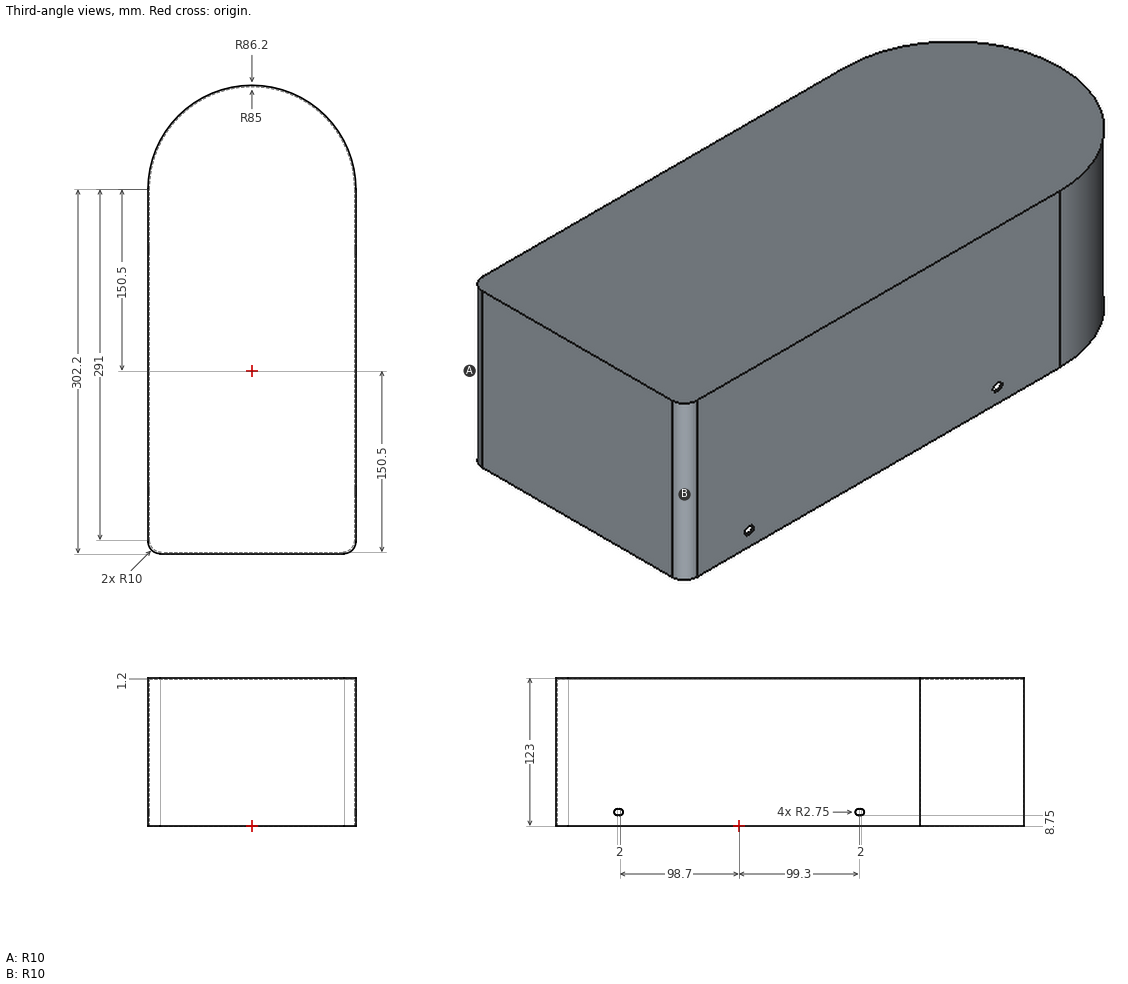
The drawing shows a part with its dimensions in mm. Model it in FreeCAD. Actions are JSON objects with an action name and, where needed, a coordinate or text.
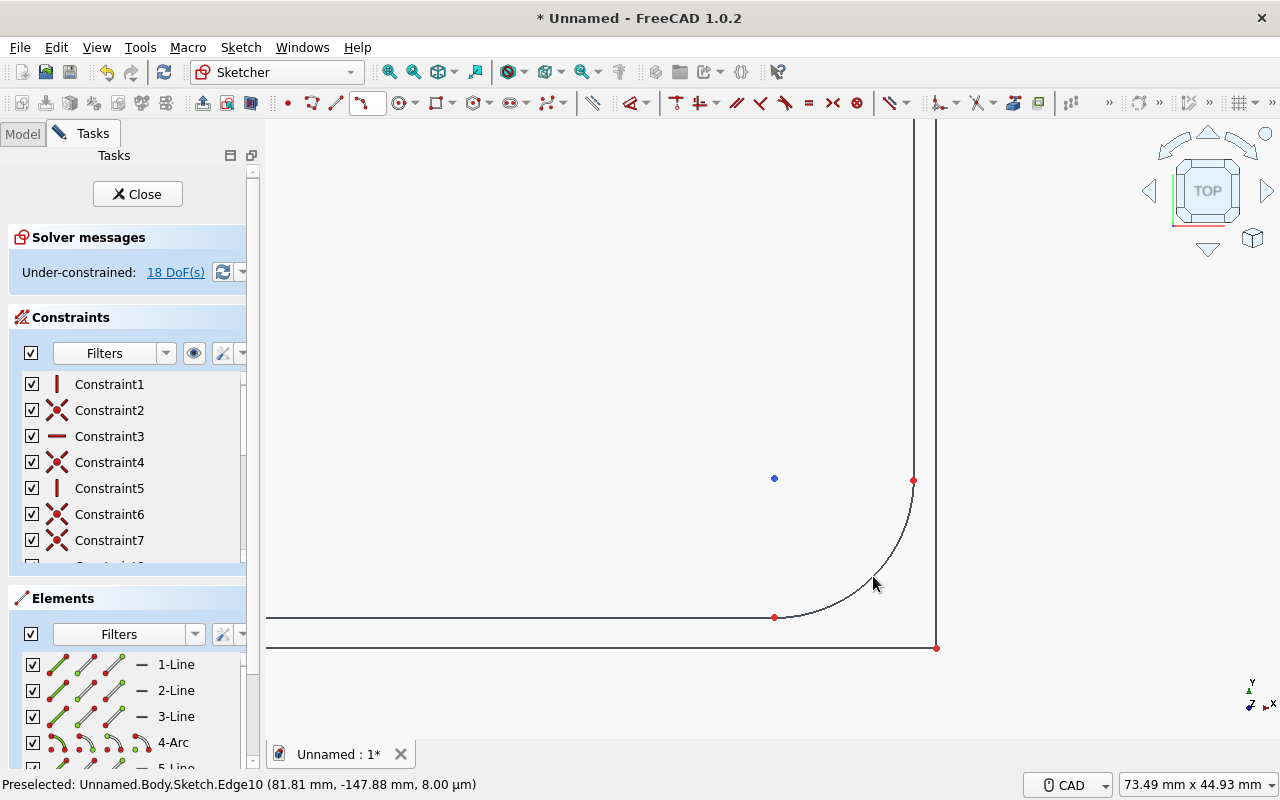
{"action": "left_click", "coordinate": [361, 618]}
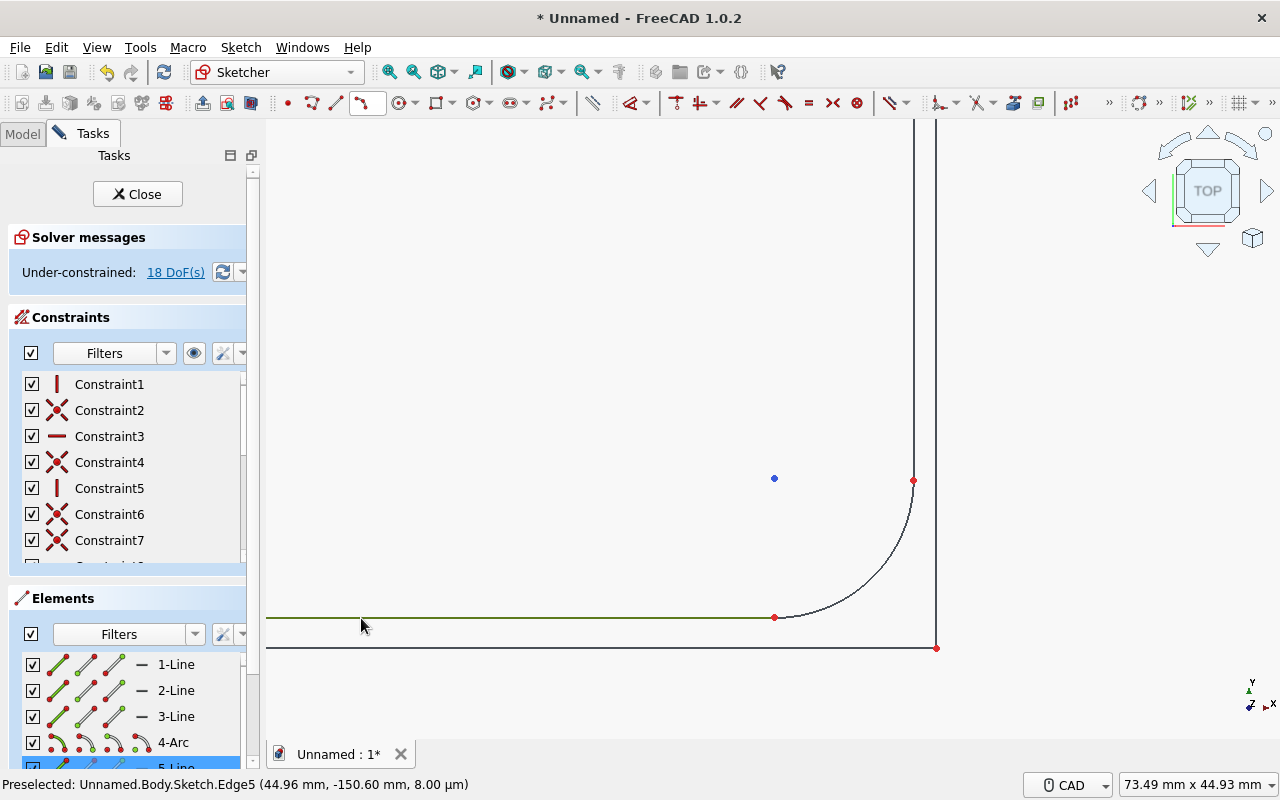
{"action": "scroll", "coordinate": [782, 628], "scroll_direction": "down", "scroll_amount": 13}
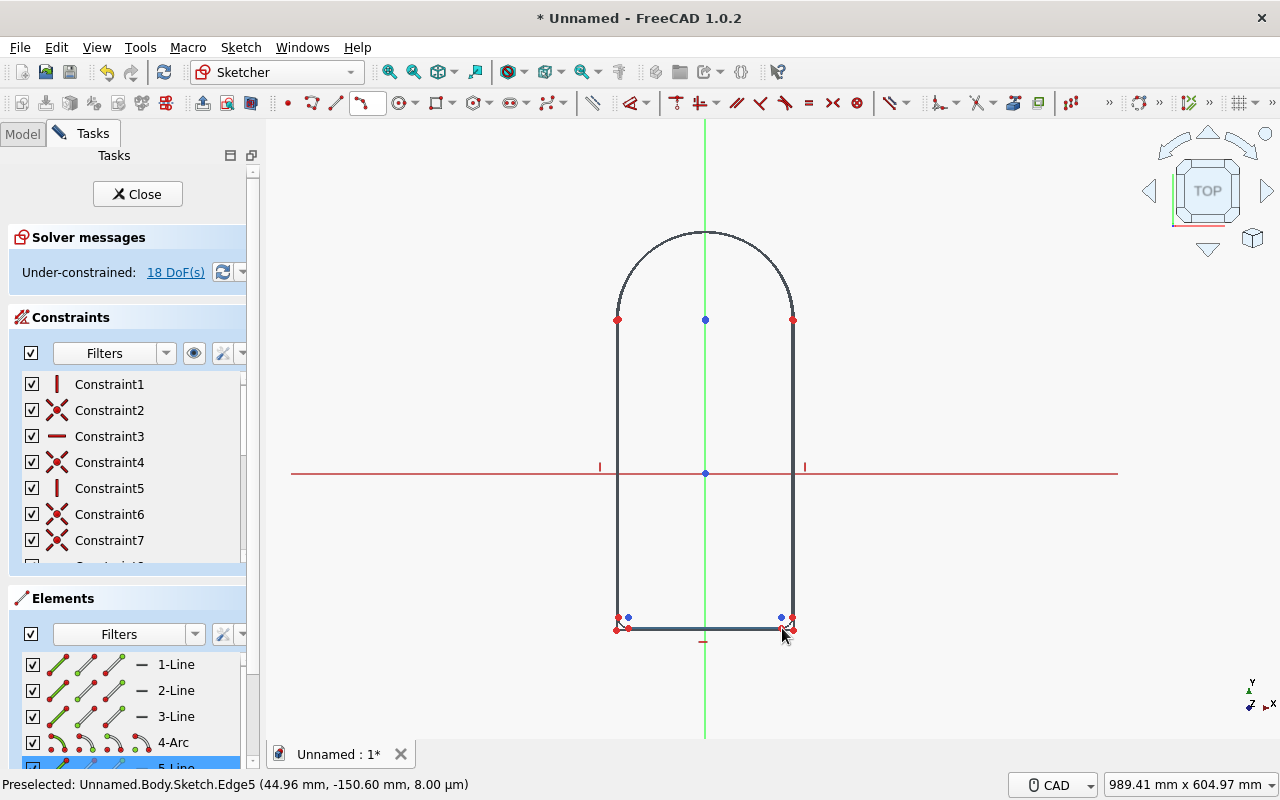
{"action": "scroll", "coordinate": [619, 622], "scroll_direction": "up", "scroll_amount": 9}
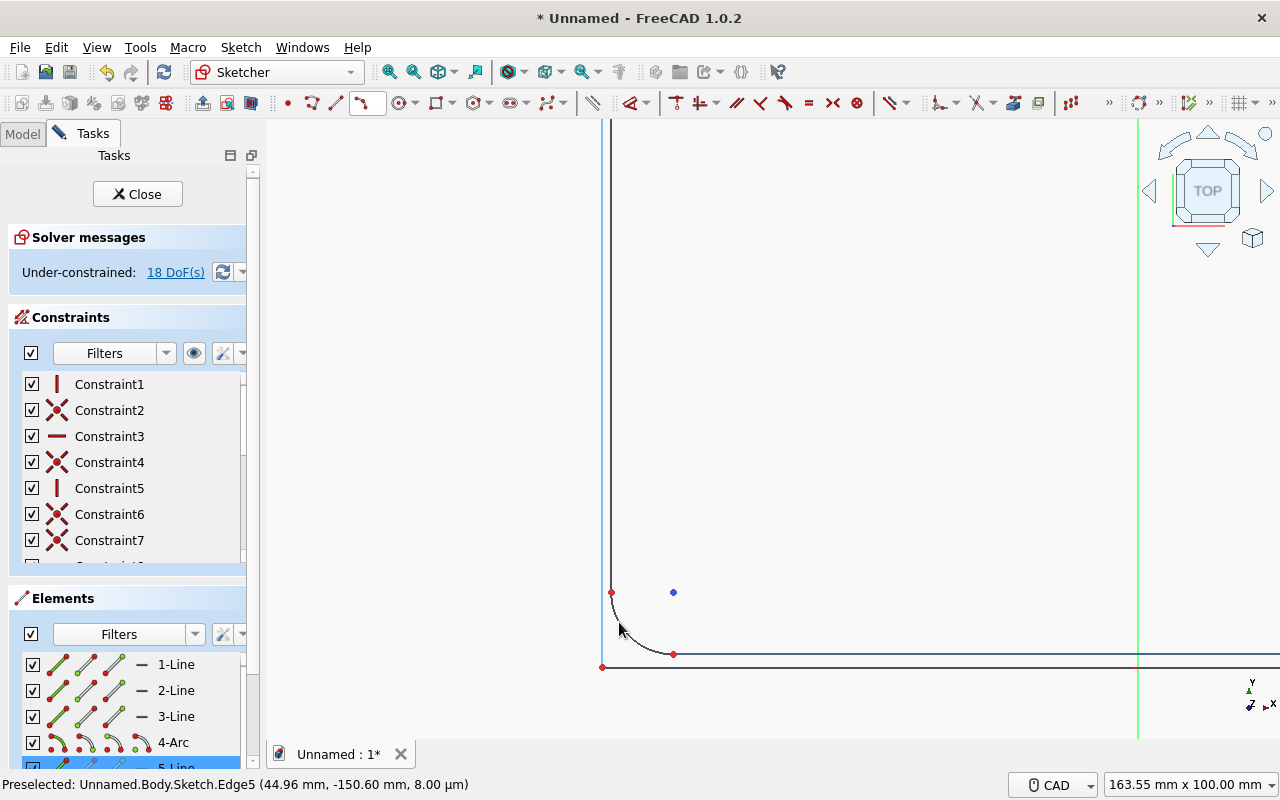
{"action": "left_click", "coordinate": [618, 620]}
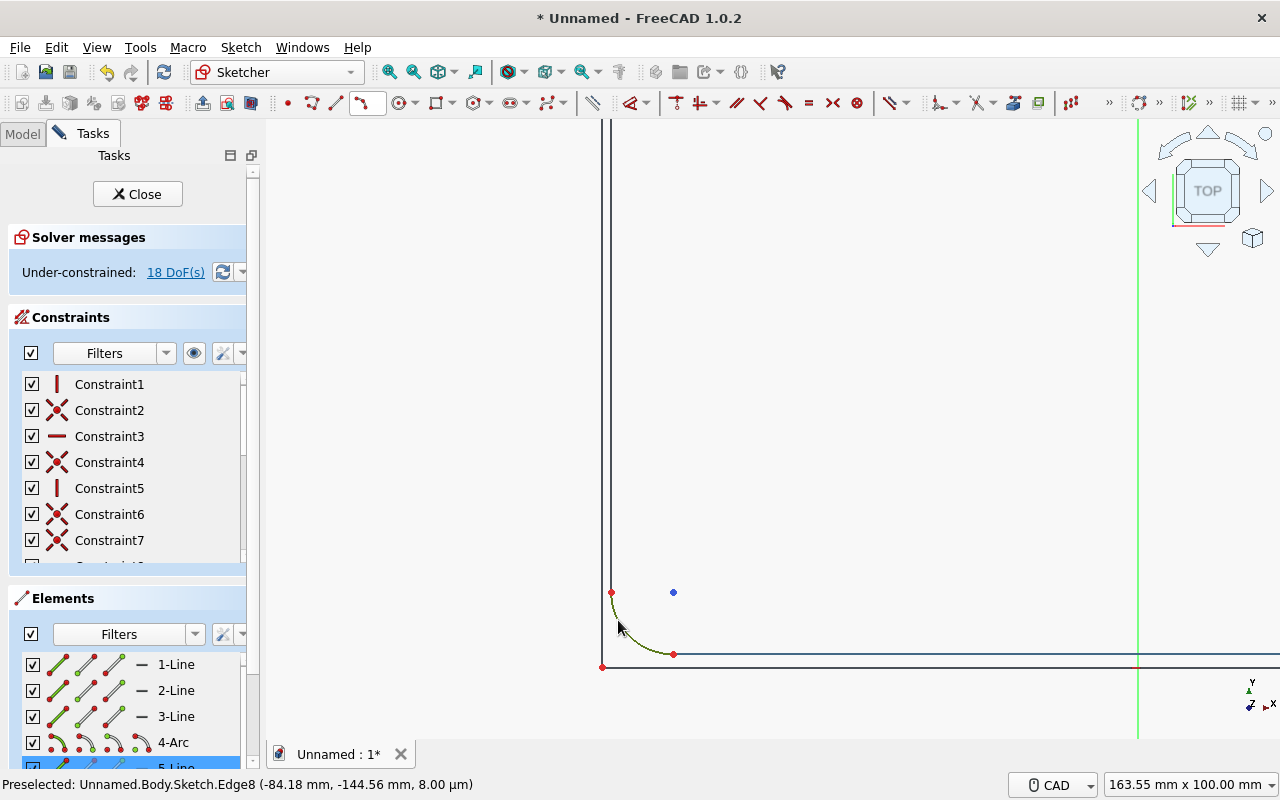
{"action": "key", "text": "t"}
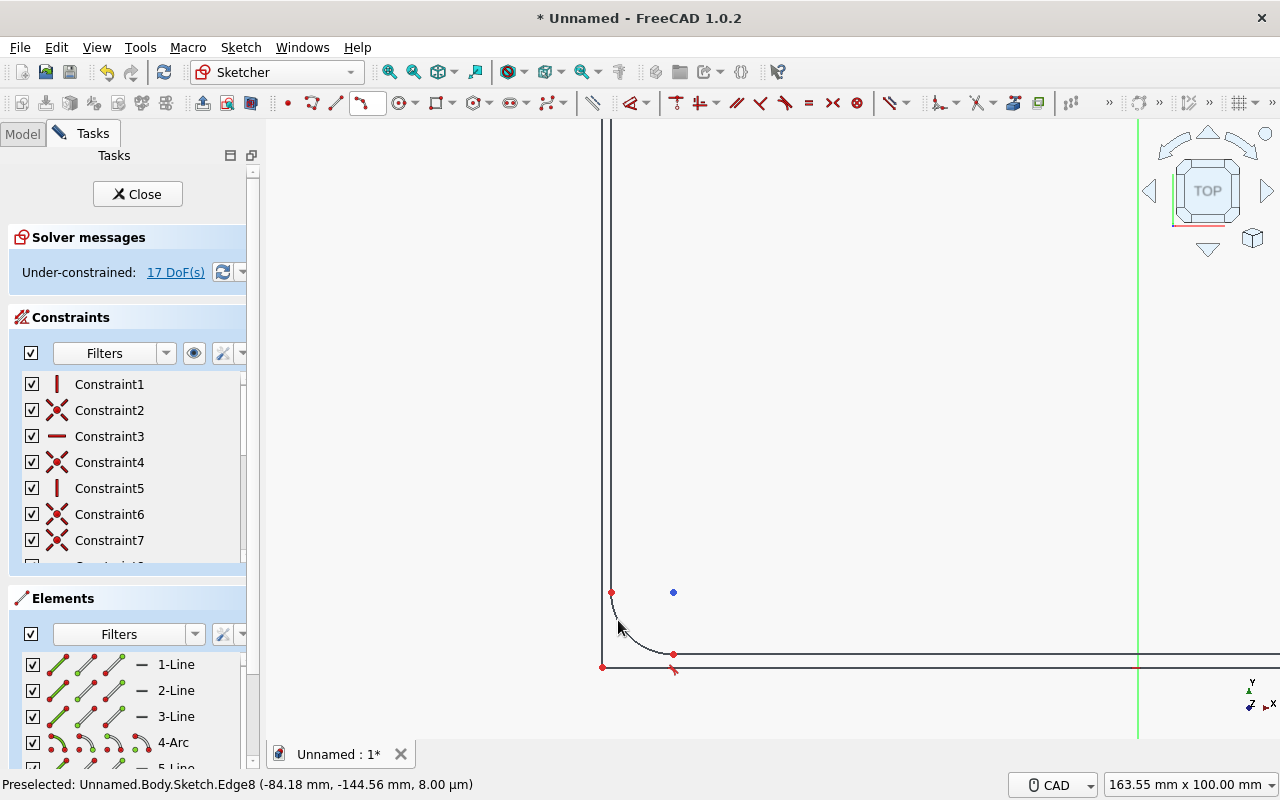
{"action": "left_click", "coordinate": [952, 654]}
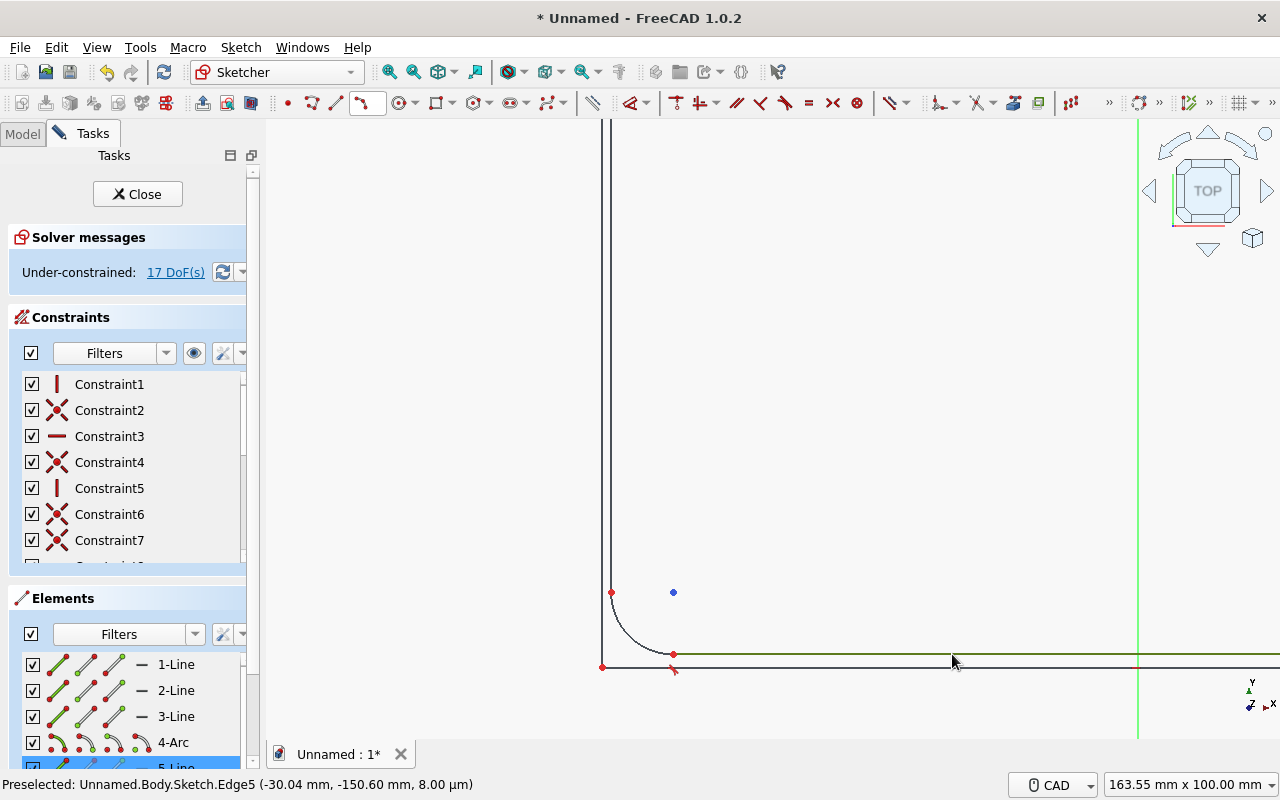
{"action": "scroll", "coordinate": [619, 621], "scroll_direction": "down", "scroll_amount": 9}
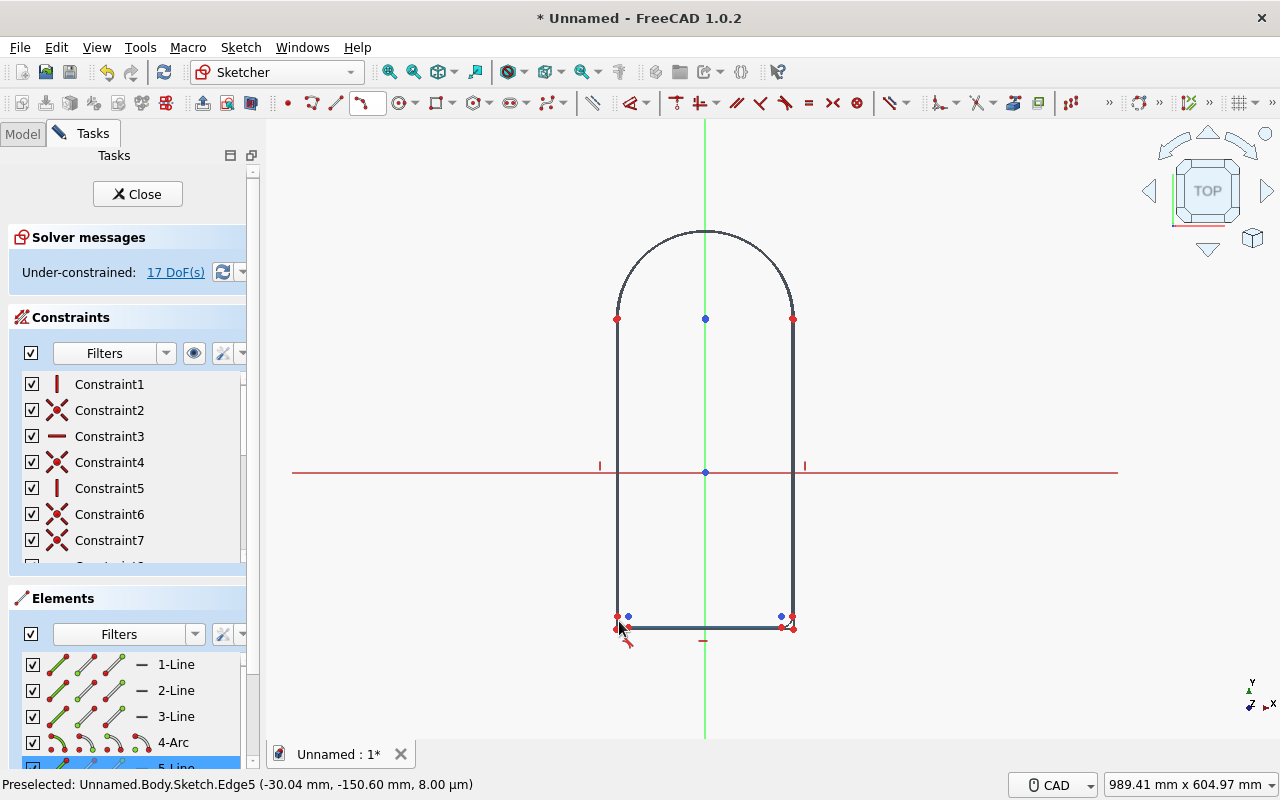
{"action": "scroll", "coordinate": [787, 626], "scroll_direction": "up", "scroll_amount": 8}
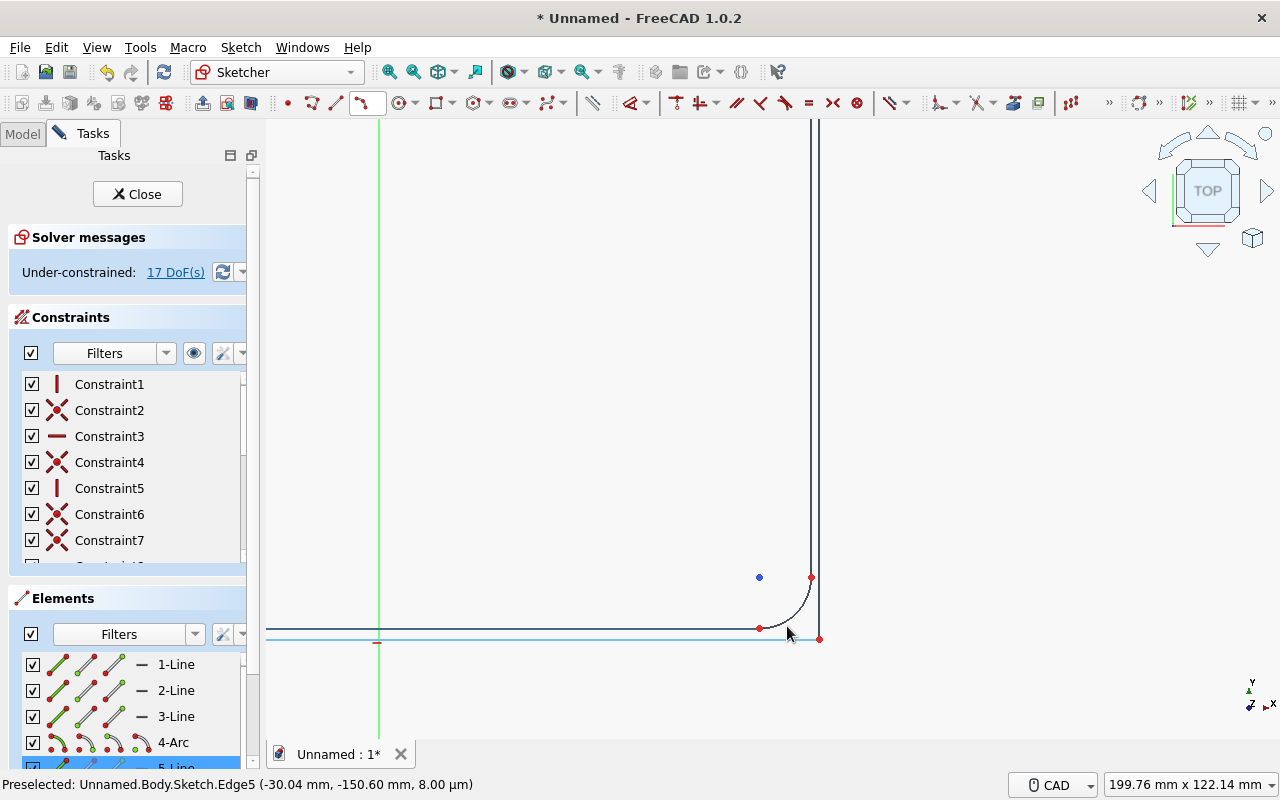
{"action": "left_click", "coordinate": [783, 623]}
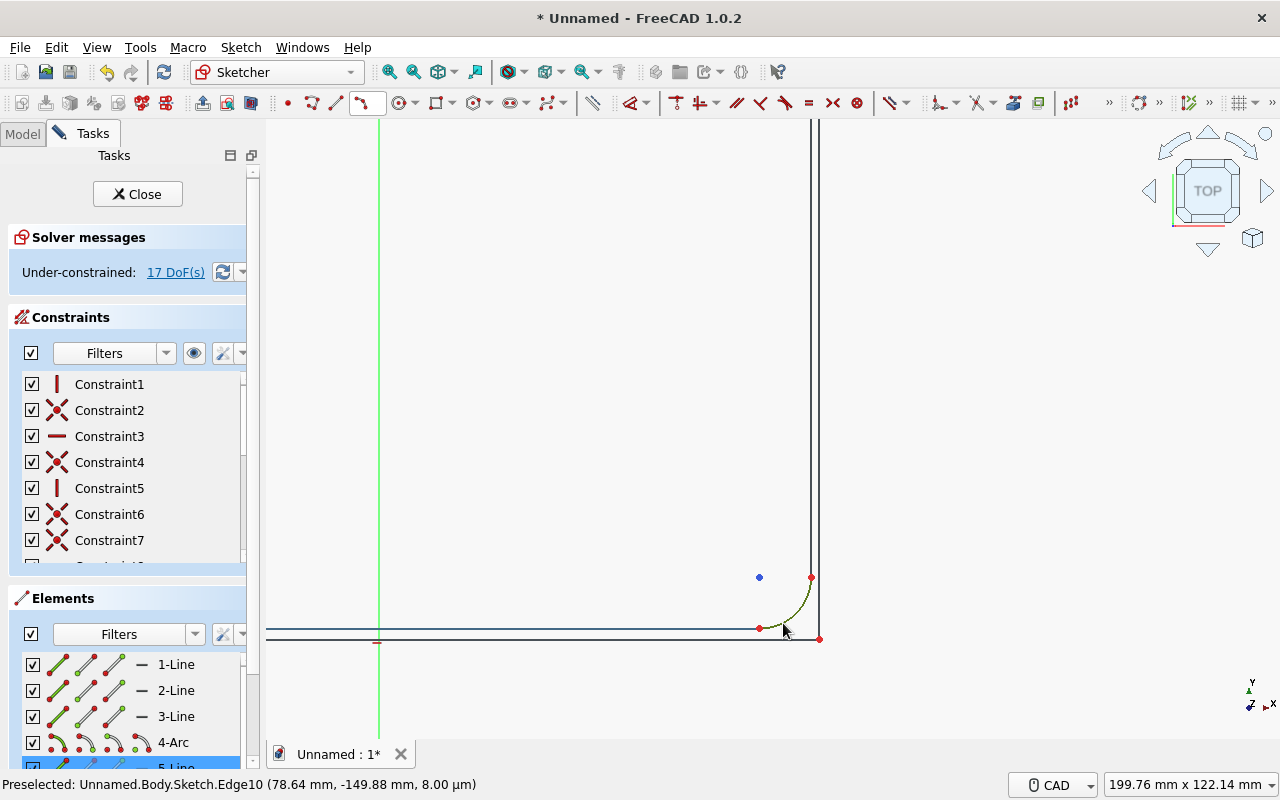
{"action": "left_click", "coordinate": [786, 104]}